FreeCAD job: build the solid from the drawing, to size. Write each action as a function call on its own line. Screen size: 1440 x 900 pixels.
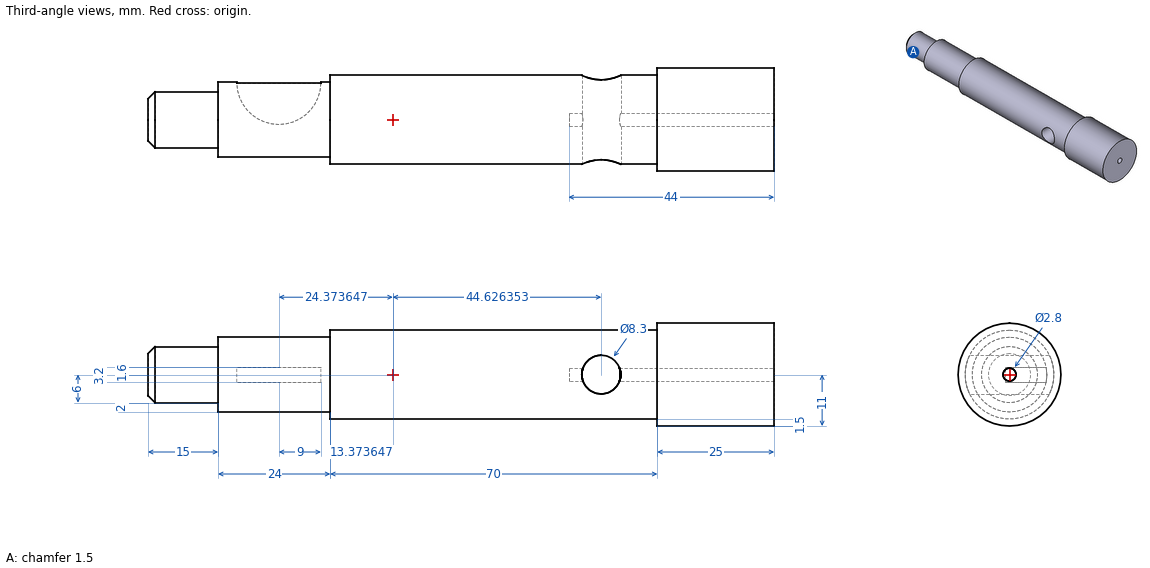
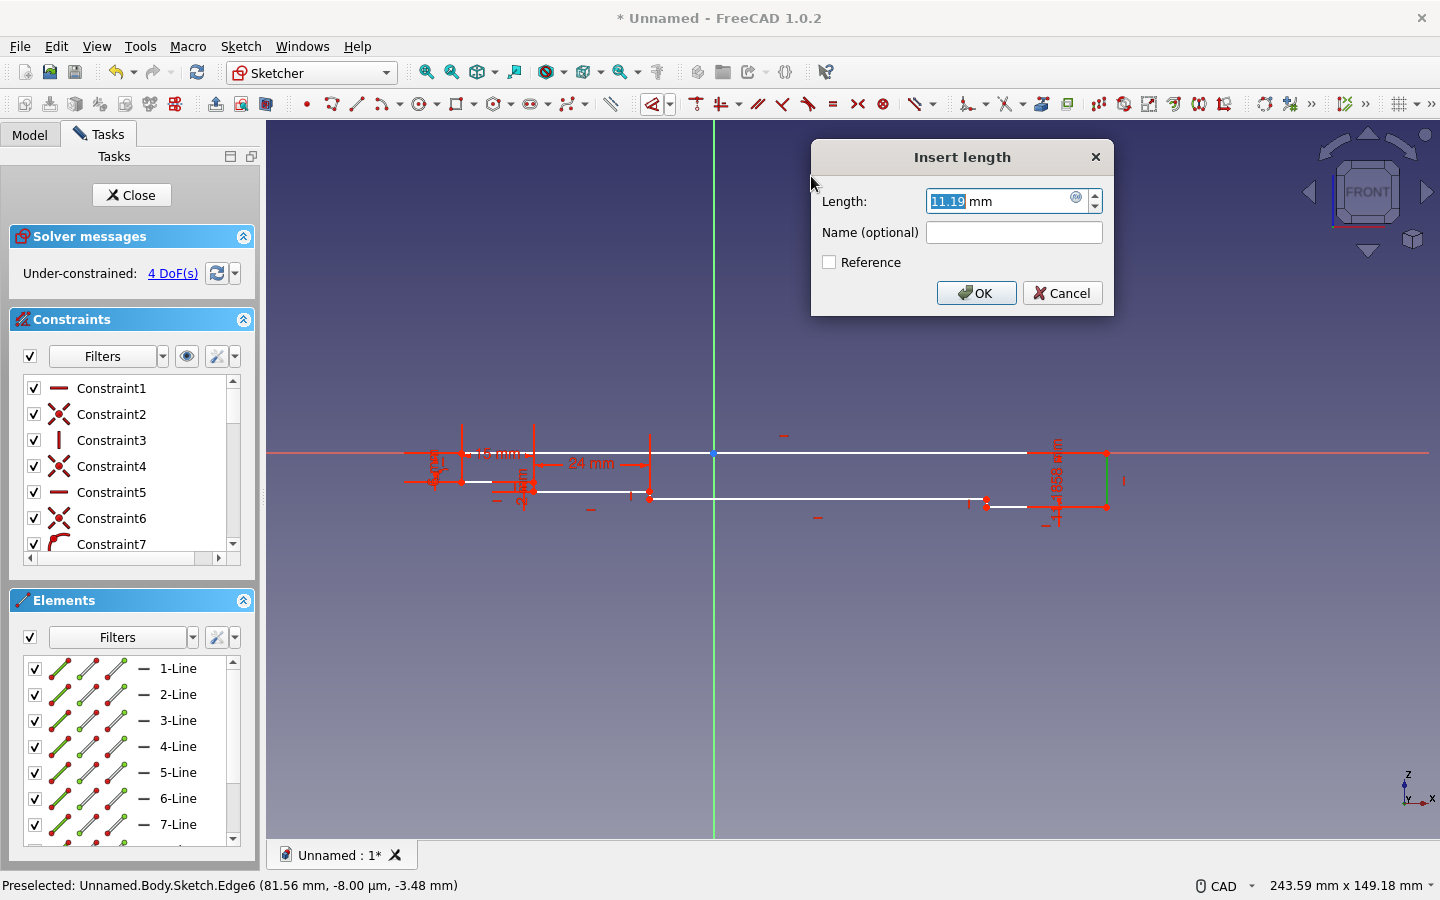
text(11)
key(Return)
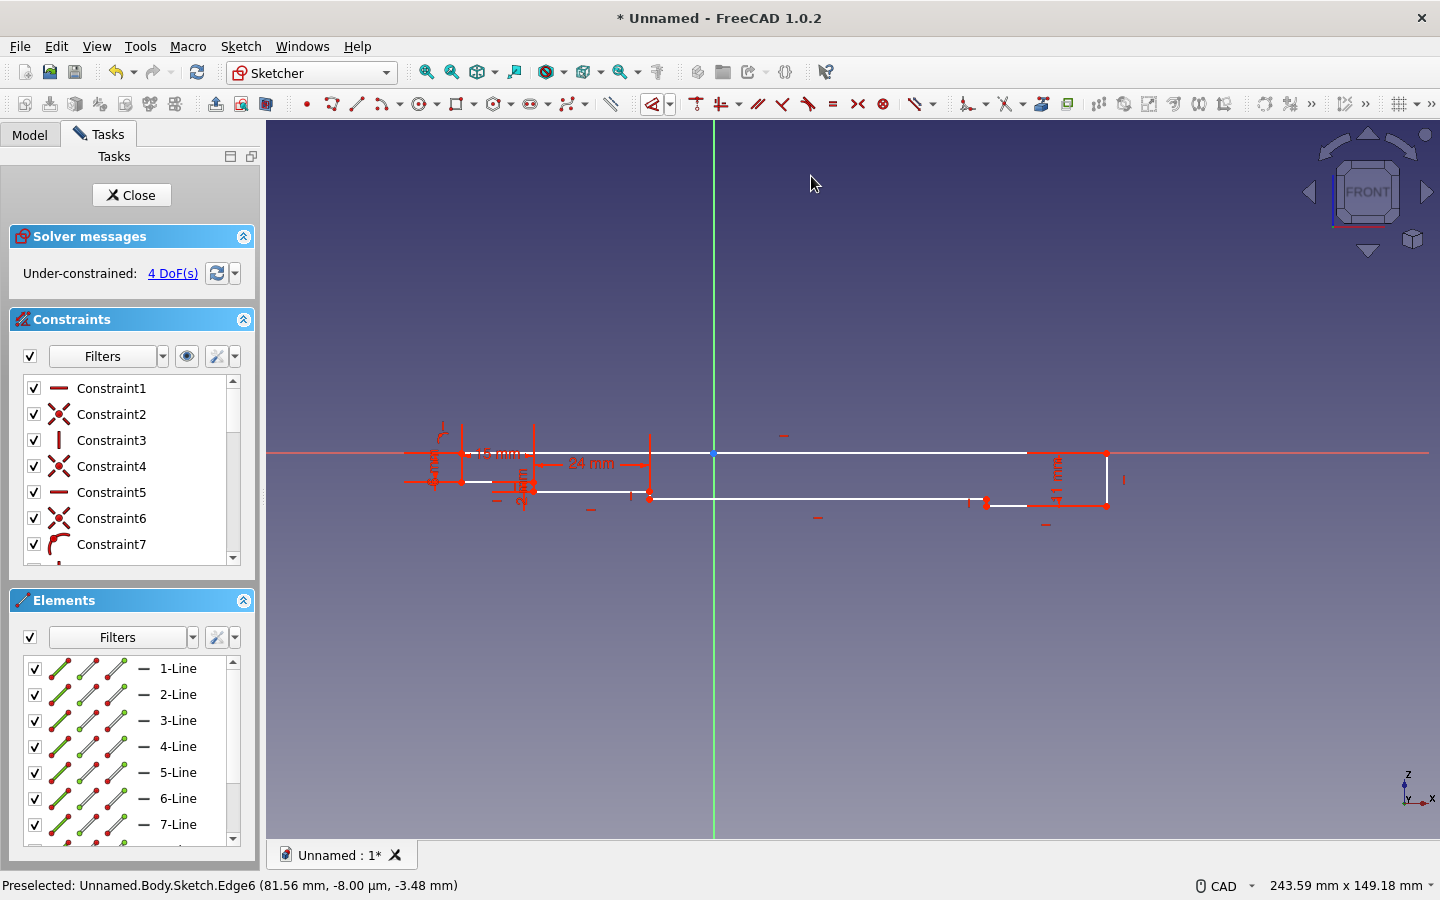
click(1071, 506)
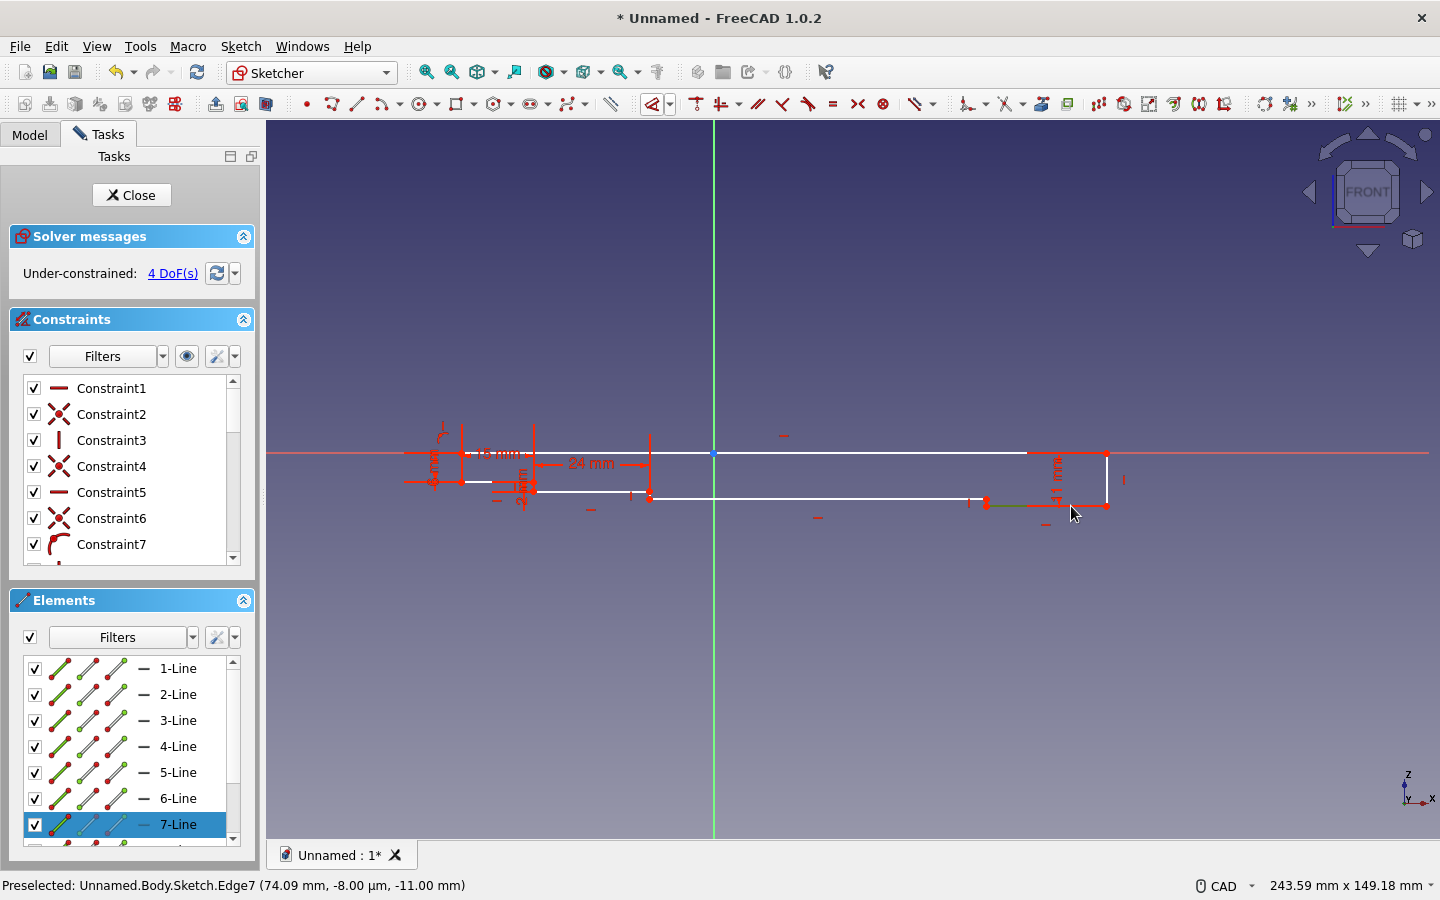
click(670, 104)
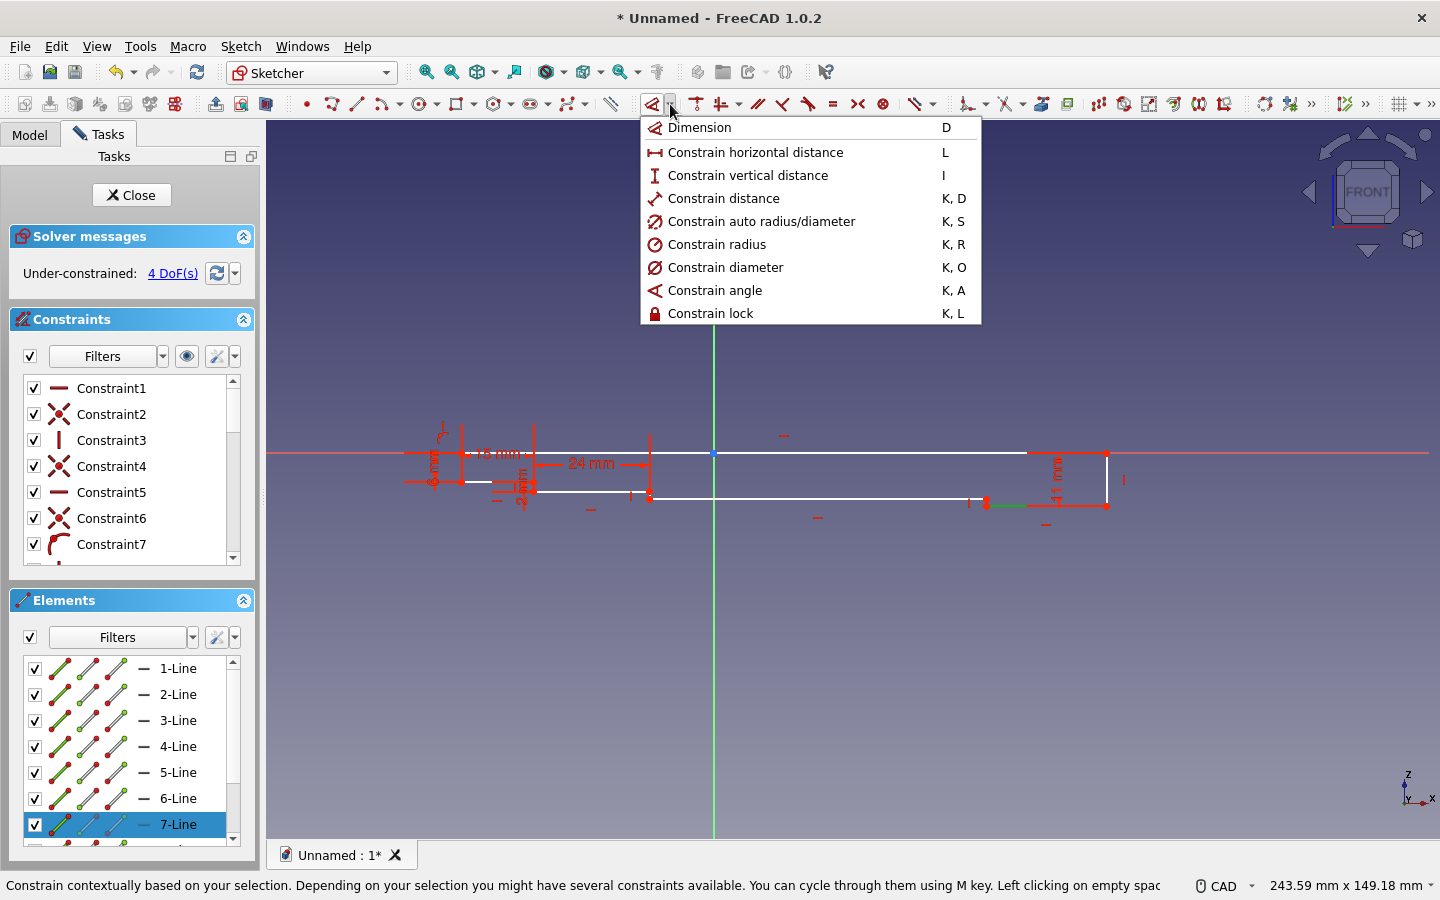
click(811, 152)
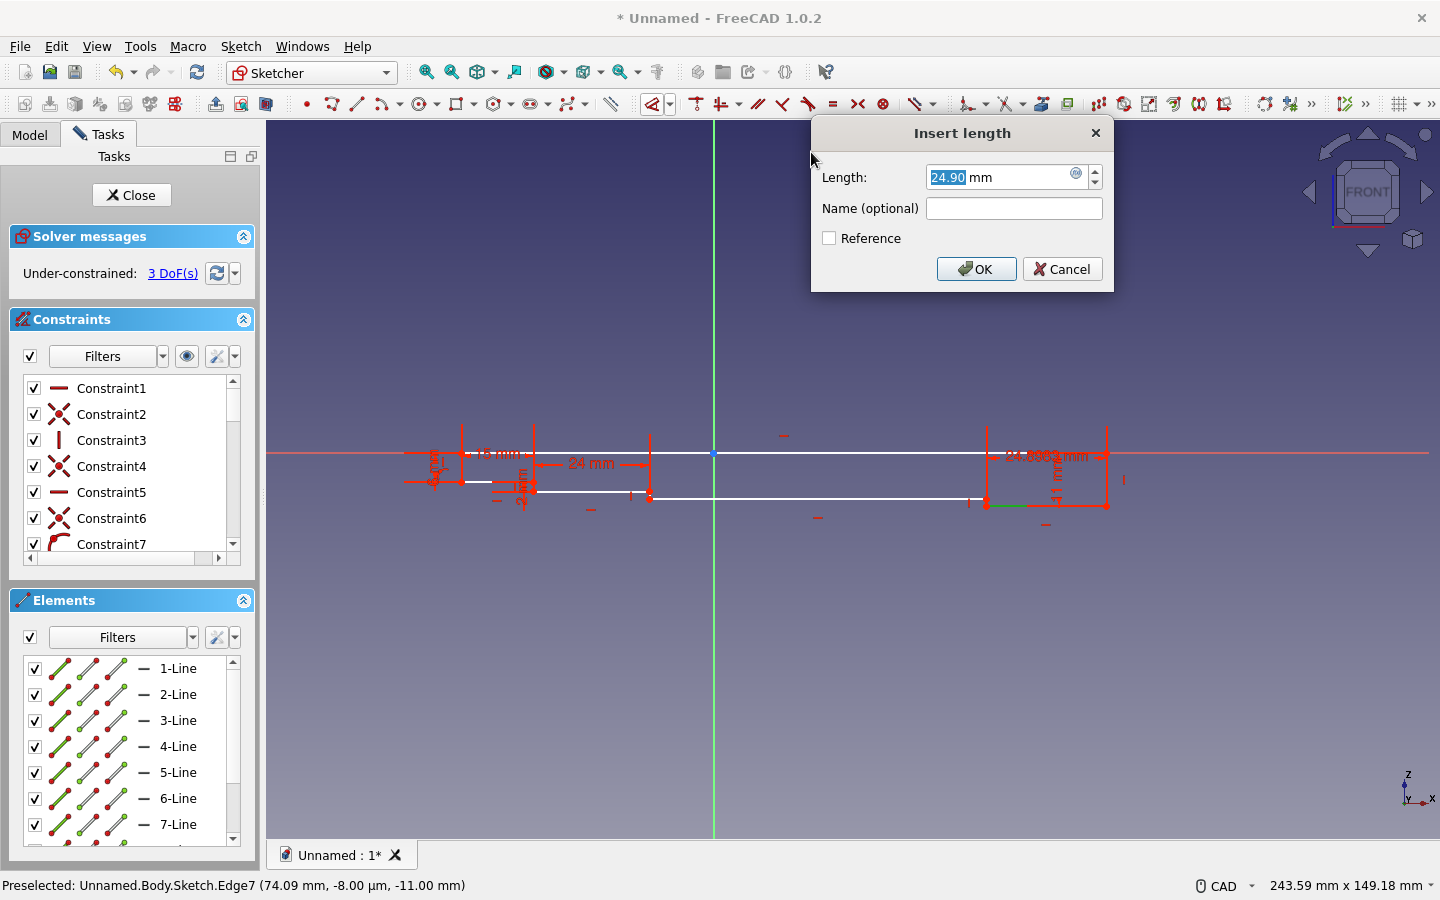
text(25)
key(Return)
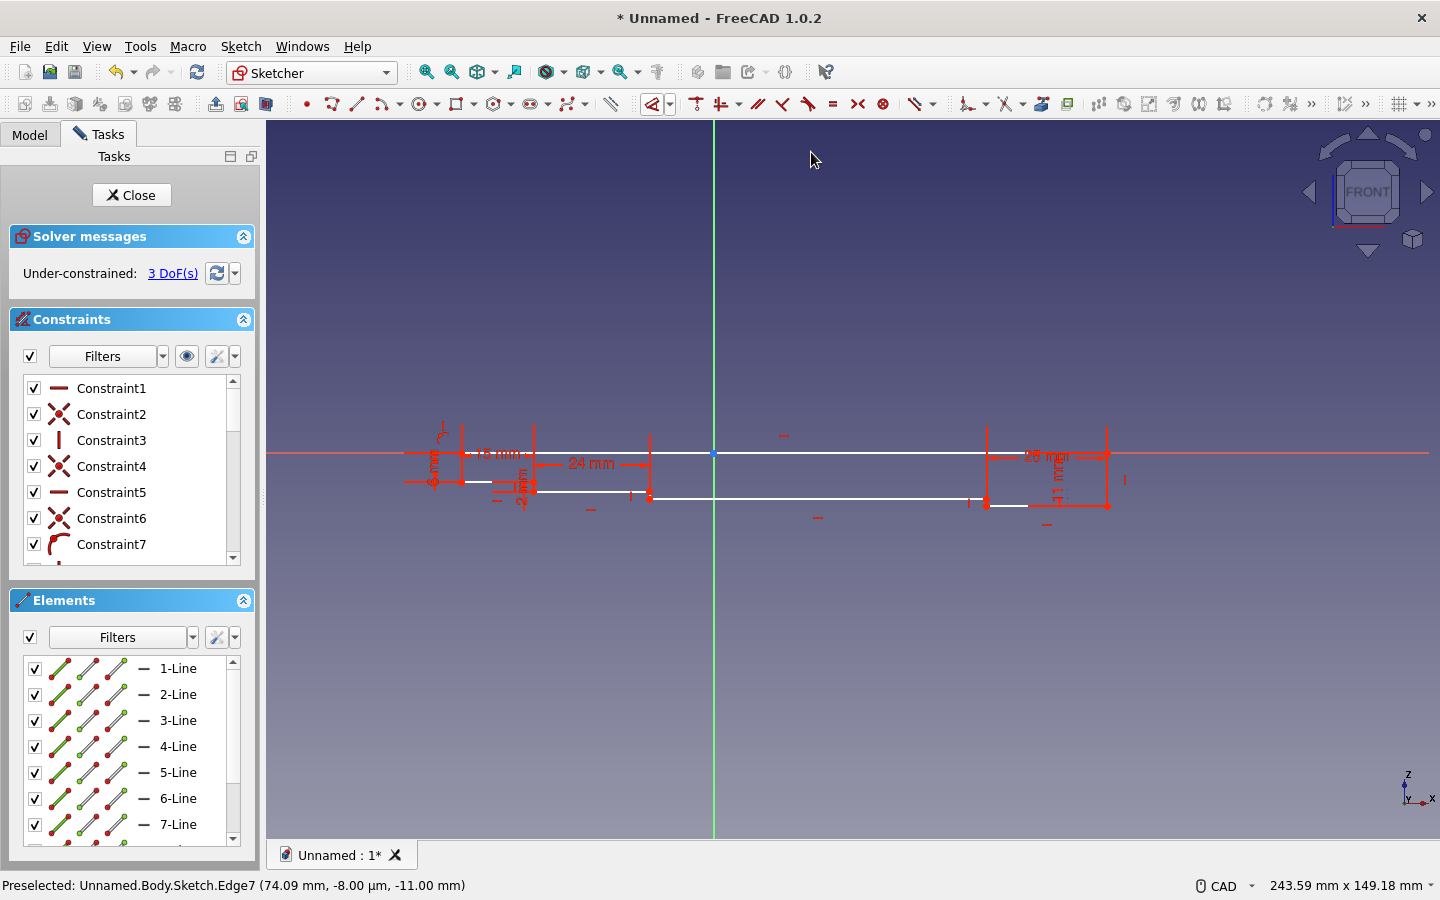
click(886, 499)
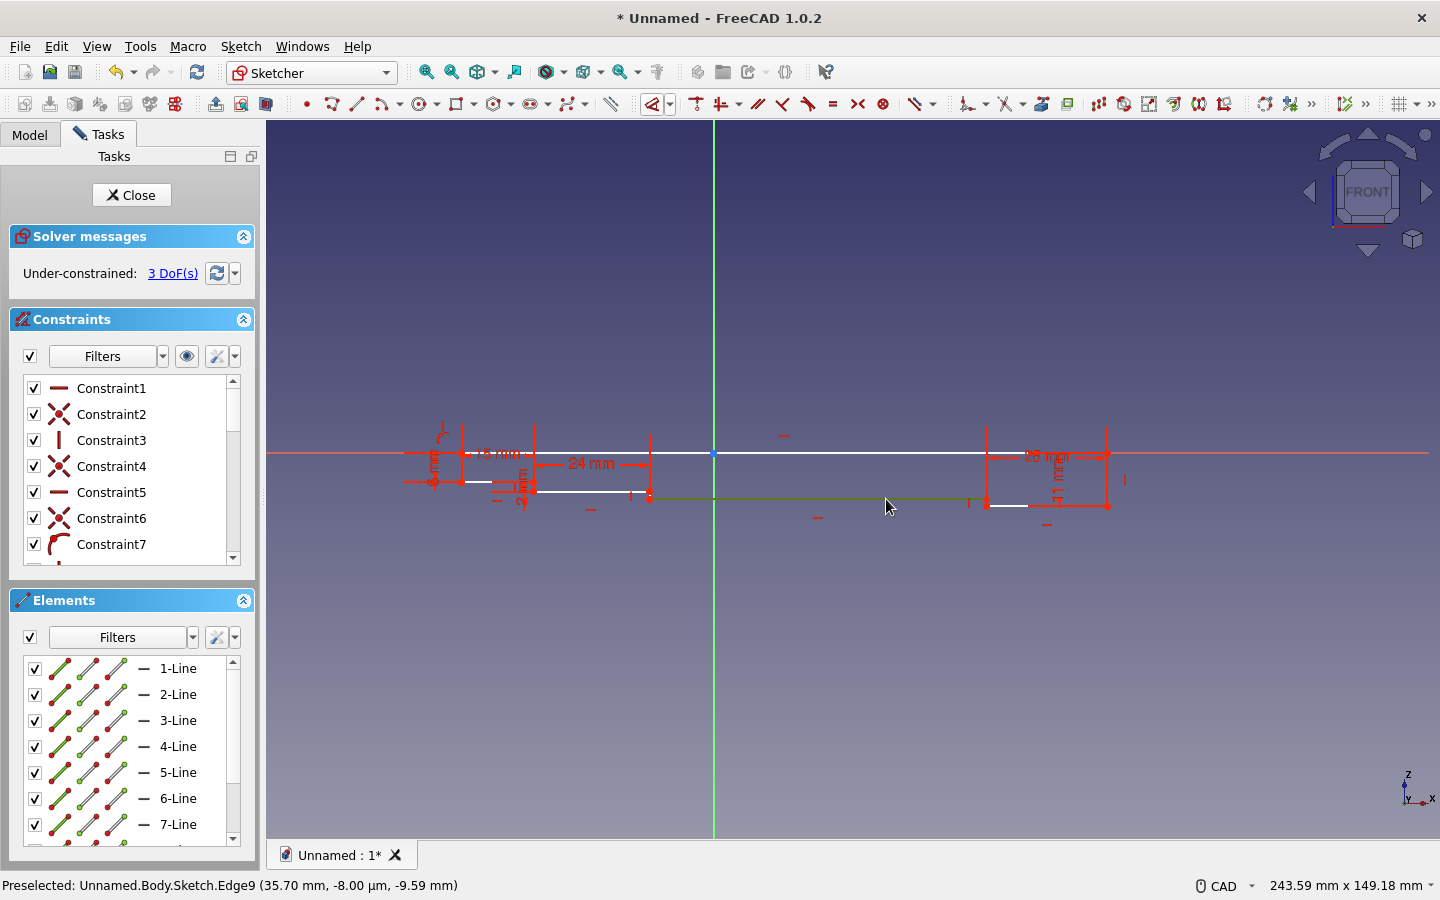
key(l)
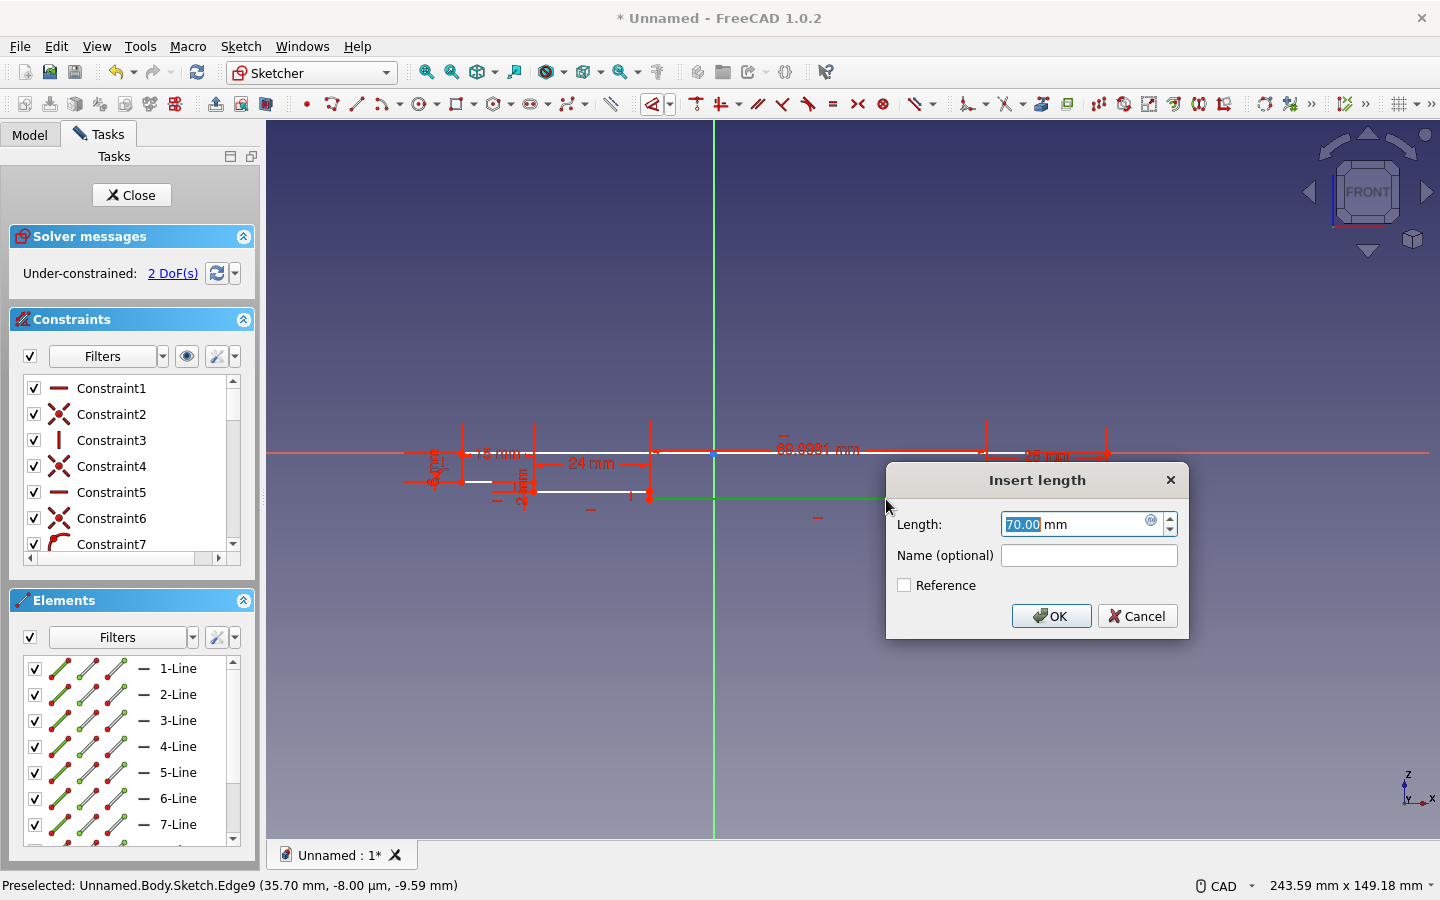
text(70)
key(Return)